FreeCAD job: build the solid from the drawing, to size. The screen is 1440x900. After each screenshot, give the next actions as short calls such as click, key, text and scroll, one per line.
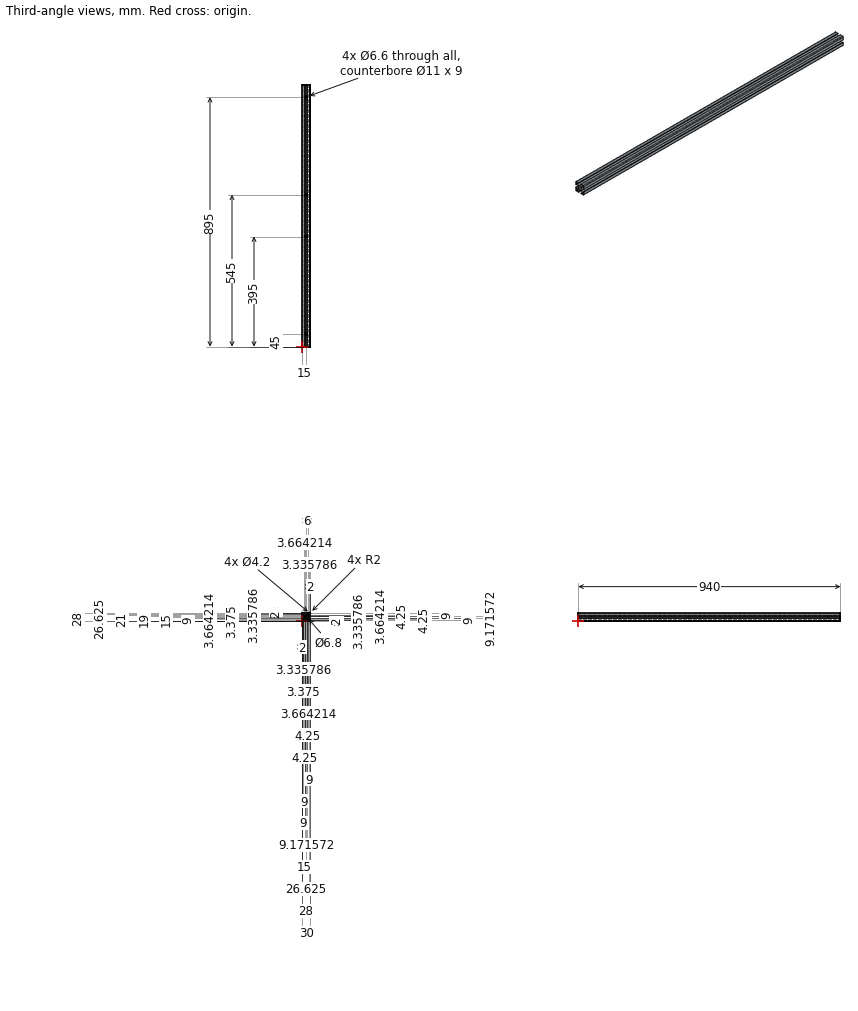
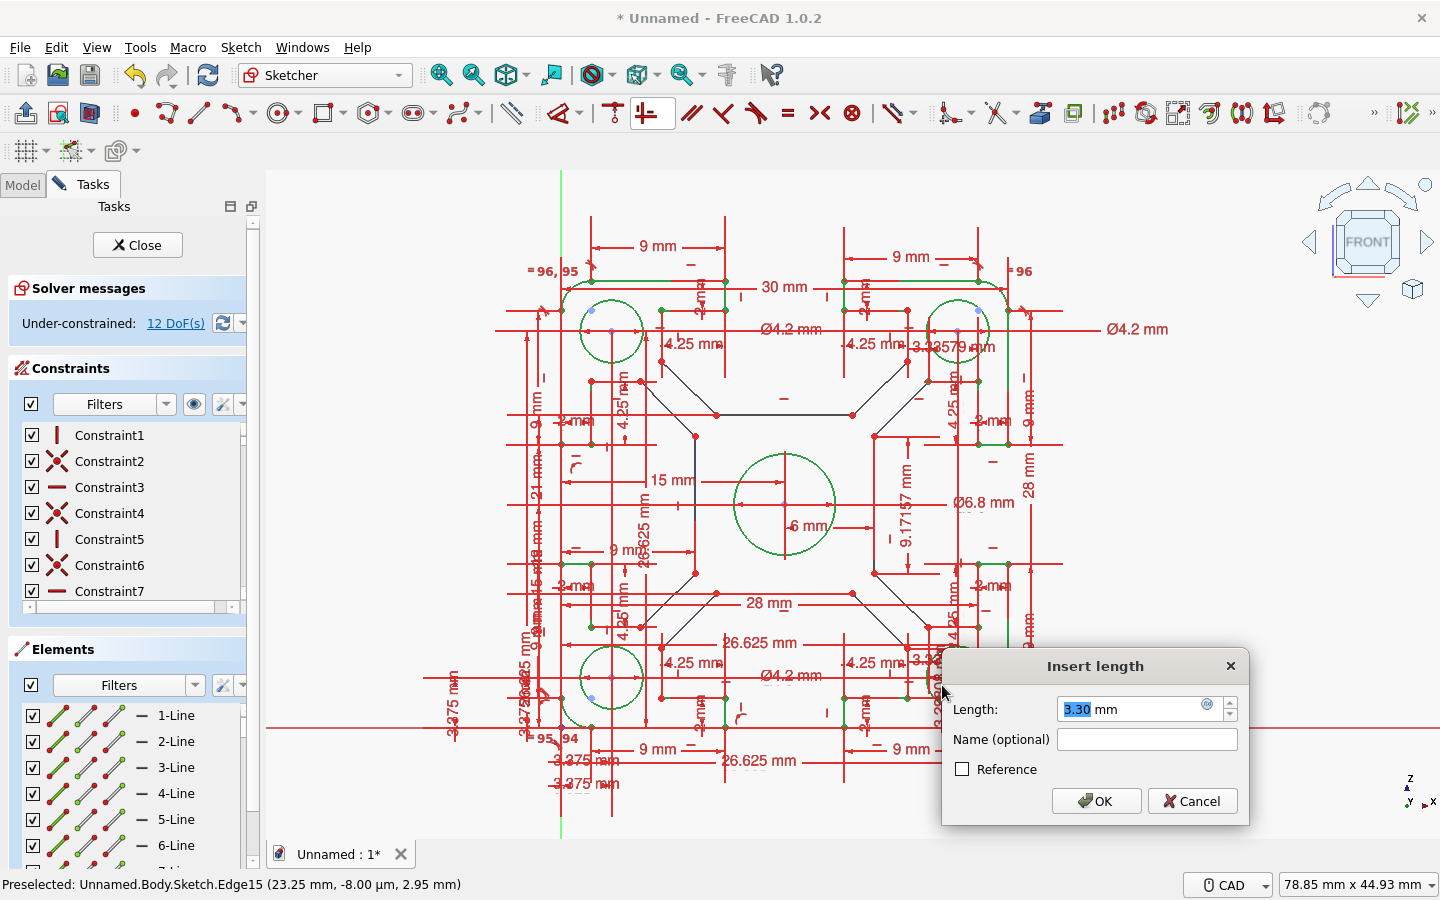
text(3.335786)
key(Return)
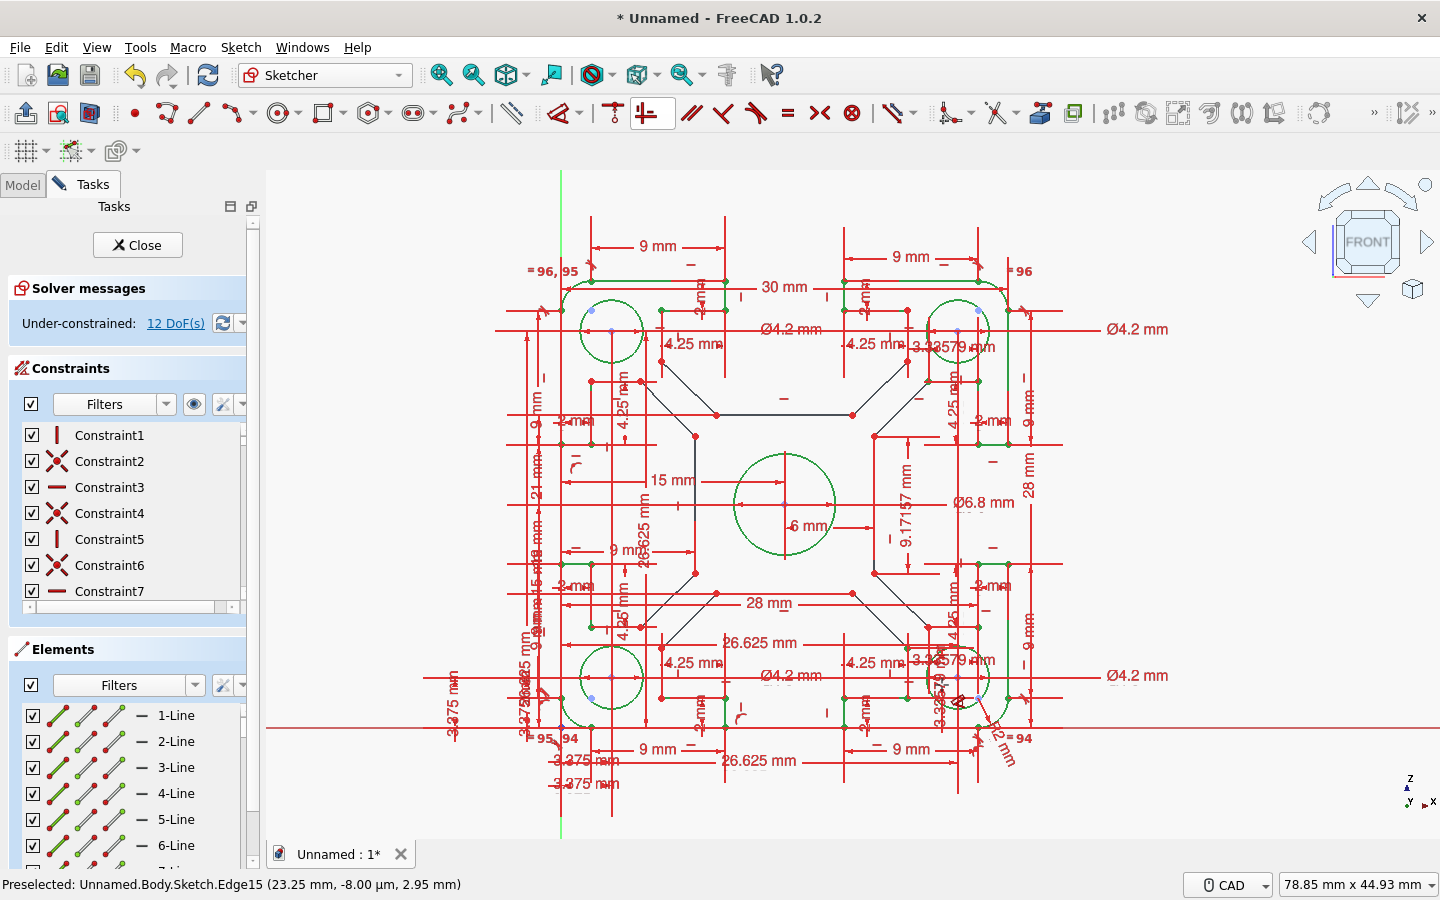
click(812, 594)
click(833, 628)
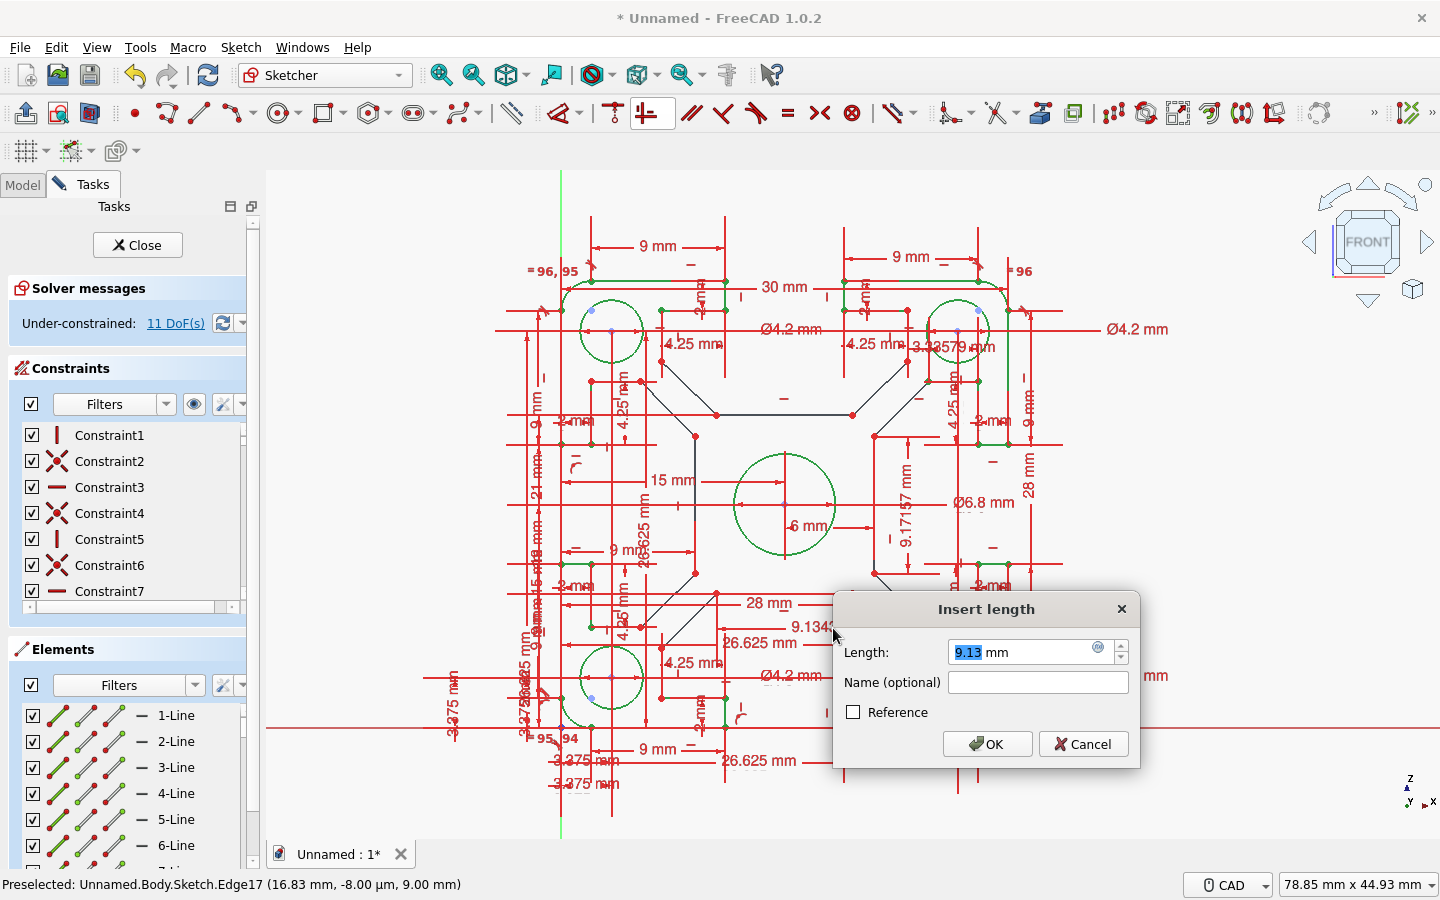
text(9.171572)
key(Return)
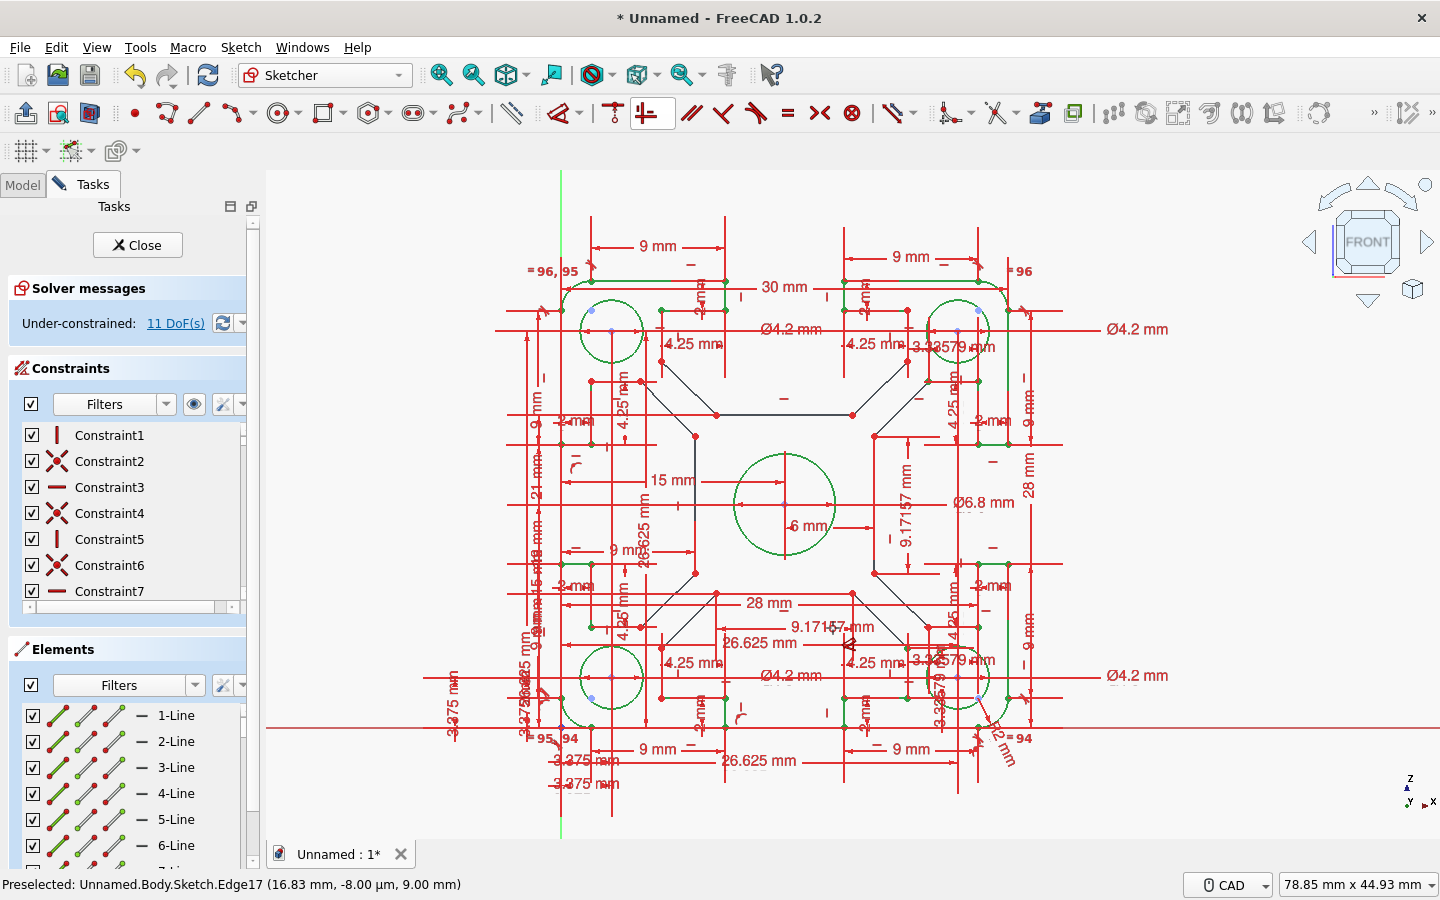
click(662, 664)
click(628, 685)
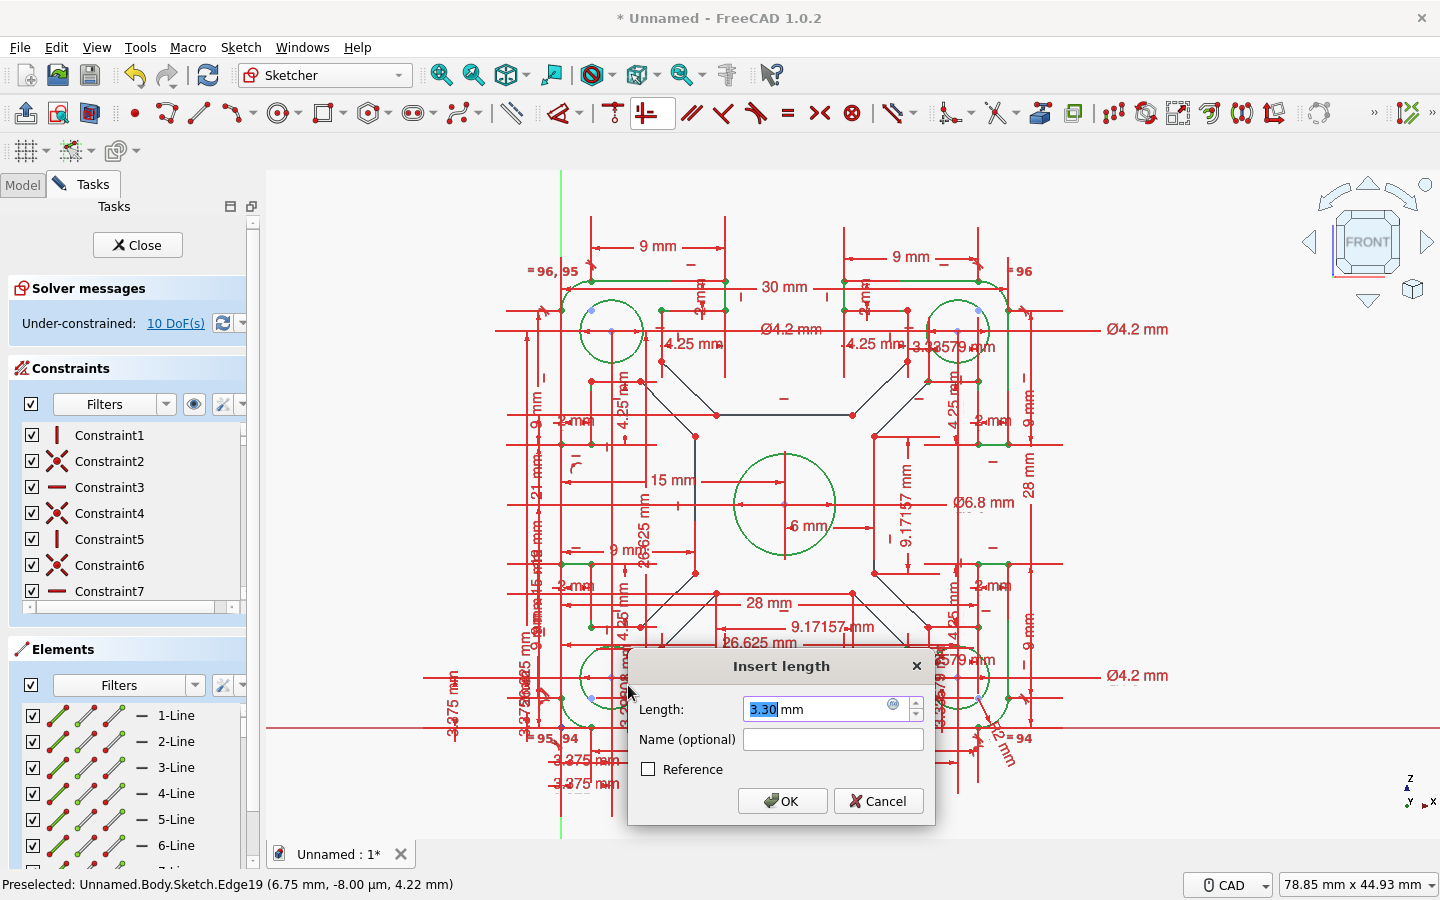
text(3.335786)
key(Return)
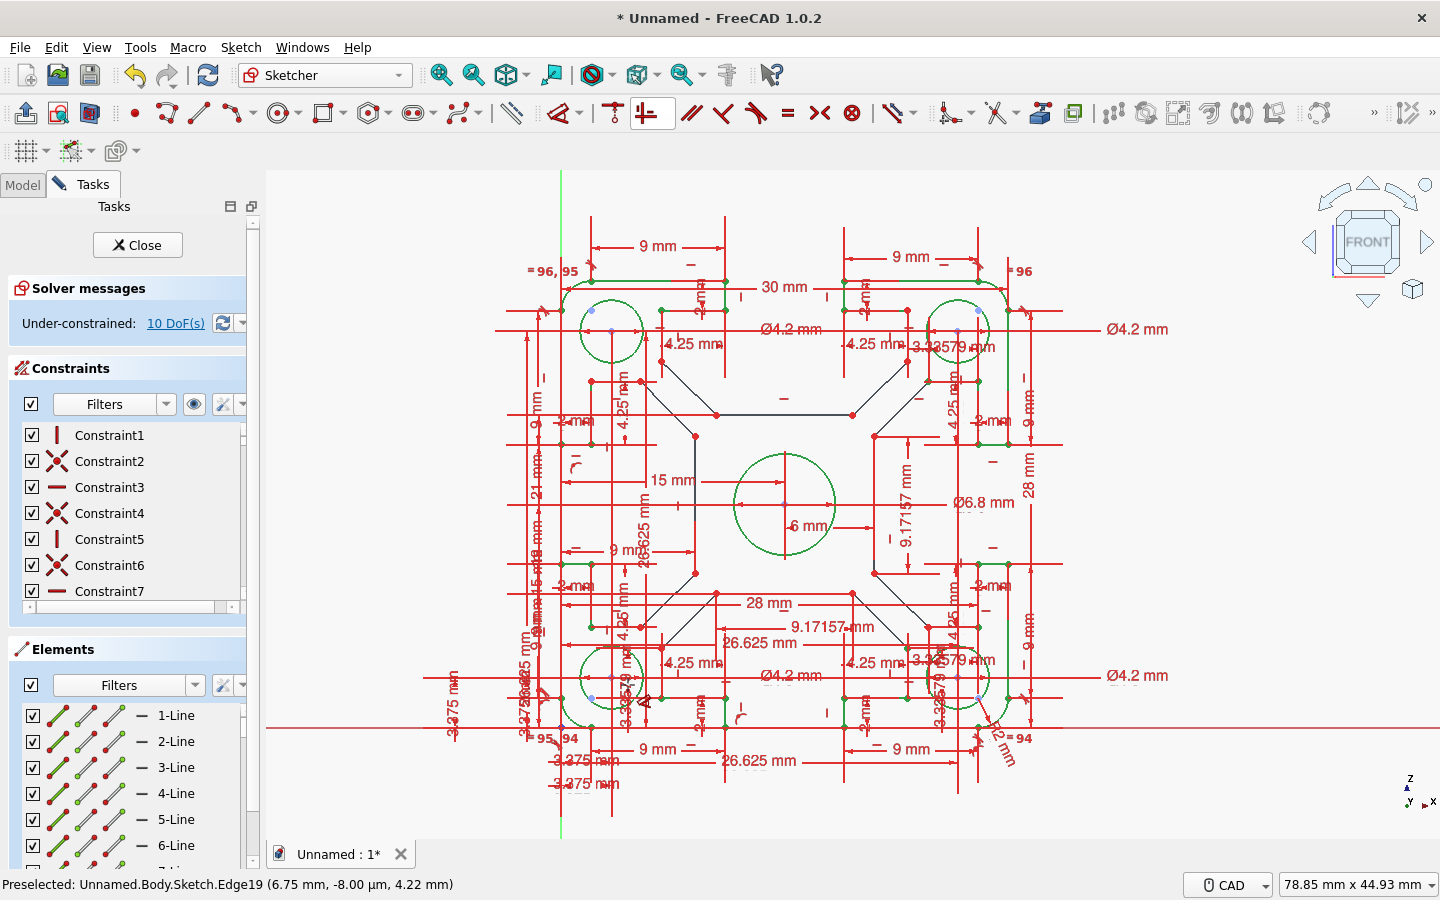
click(606, 627)
click(616, 661)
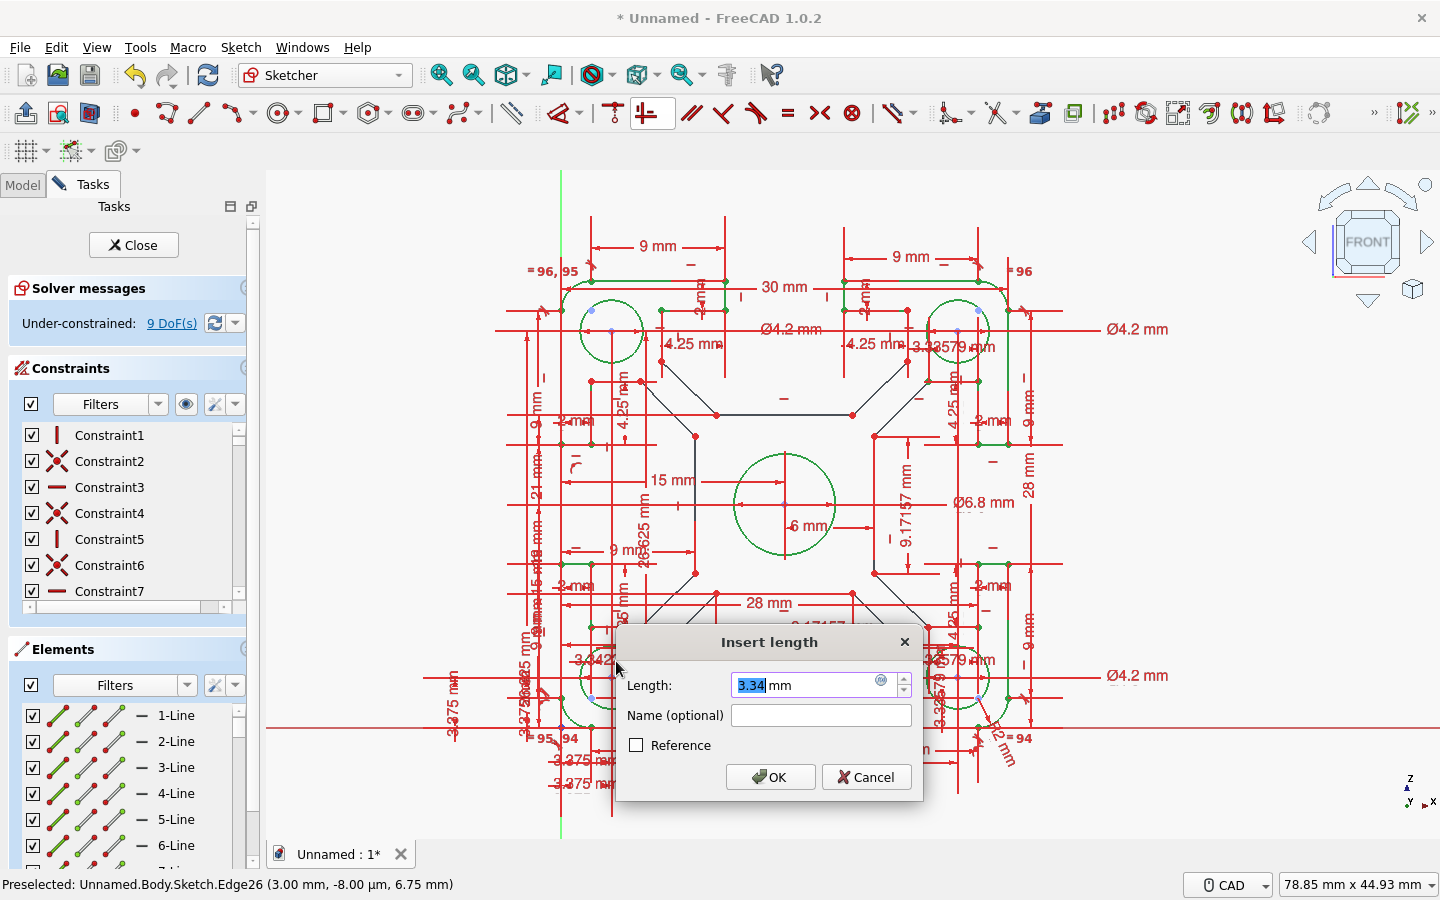
text(3.335786)
key(Return)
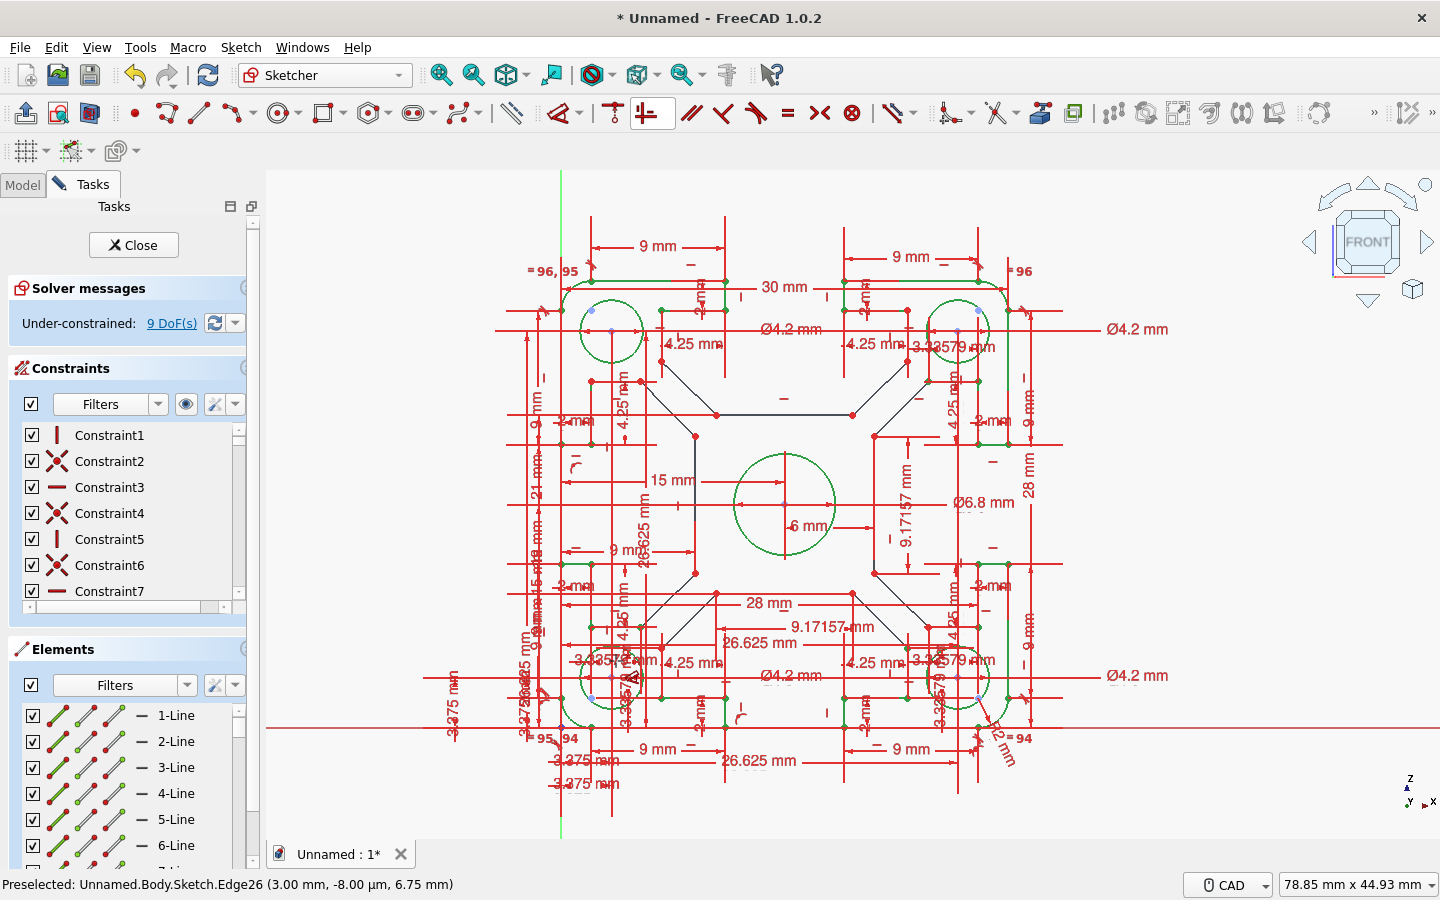
click(695, 533)
click(661, 505)